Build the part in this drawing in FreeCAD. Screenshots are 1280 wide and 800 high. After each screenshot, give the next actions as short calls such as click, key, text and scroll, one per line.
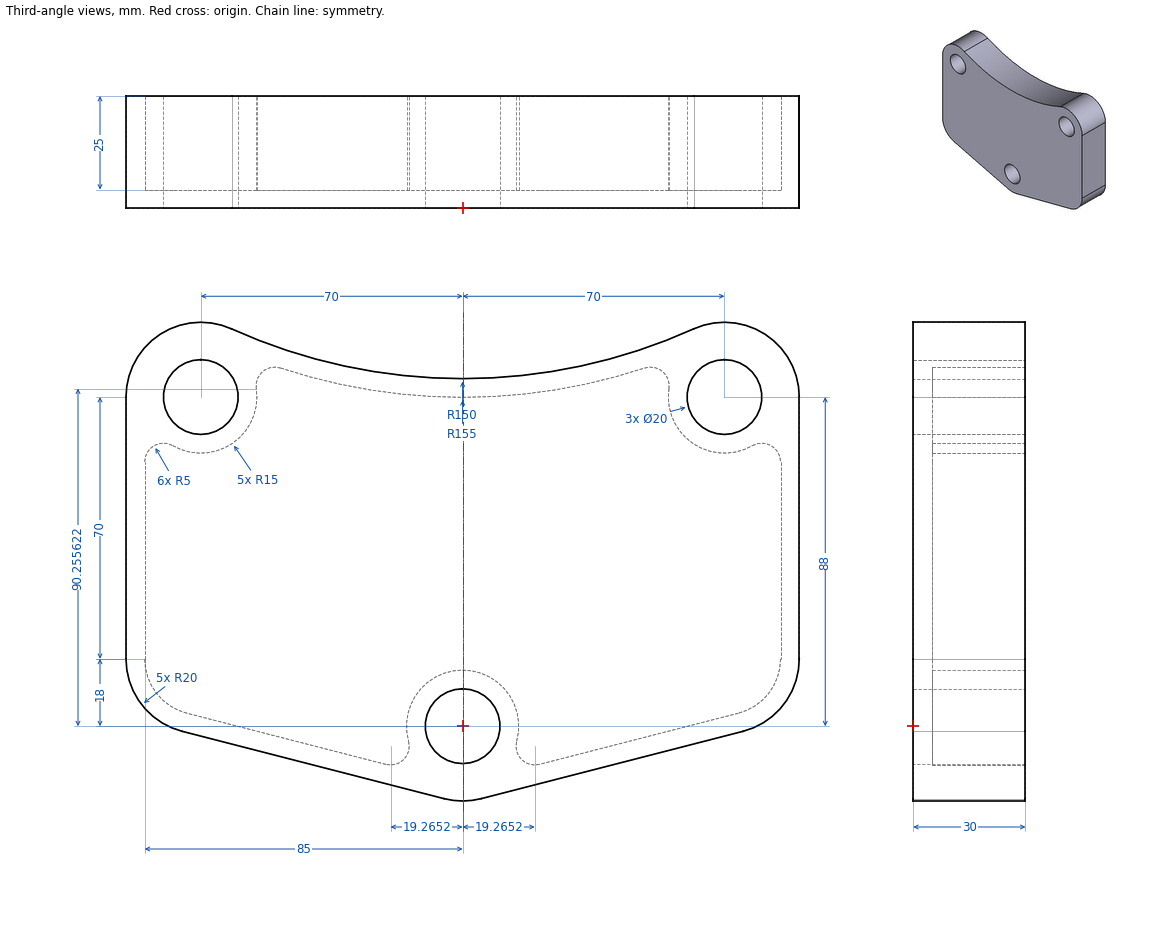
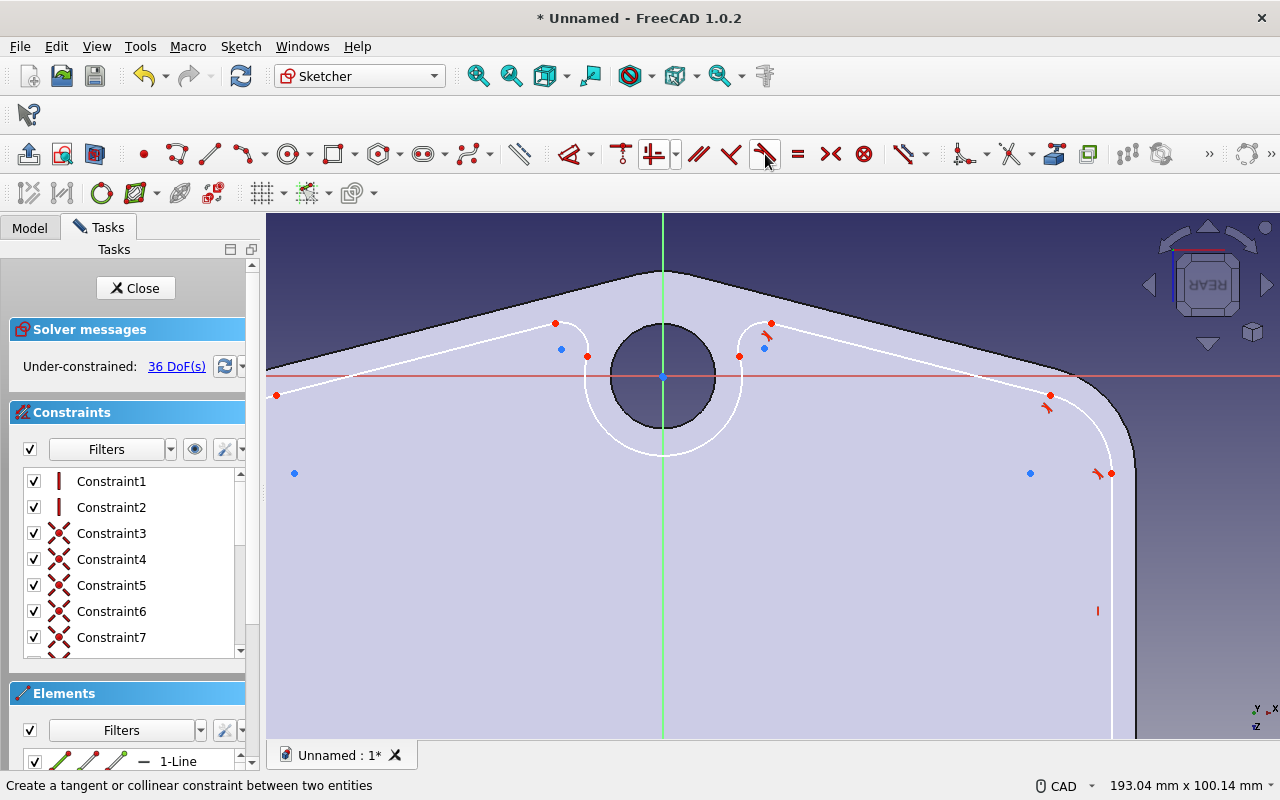
click(471, 345)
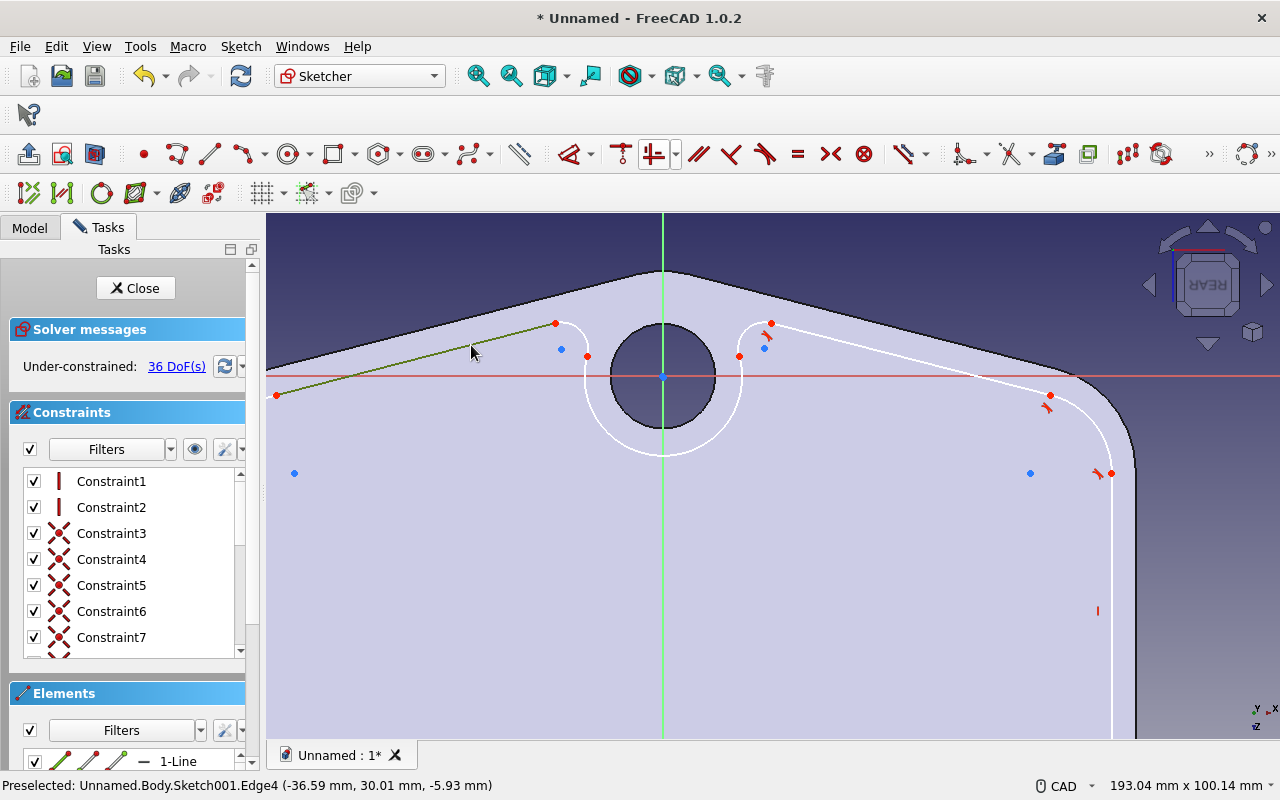
click(587, 340)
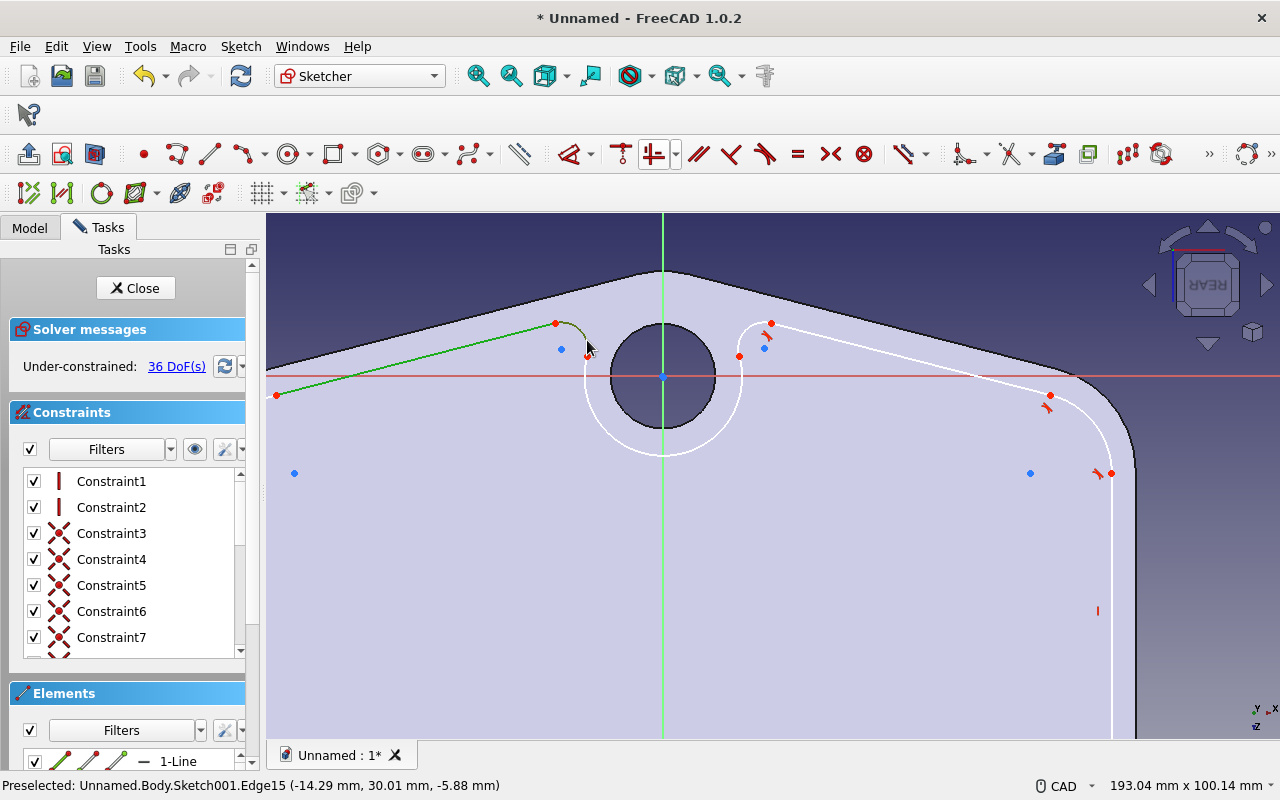
click(765, 154)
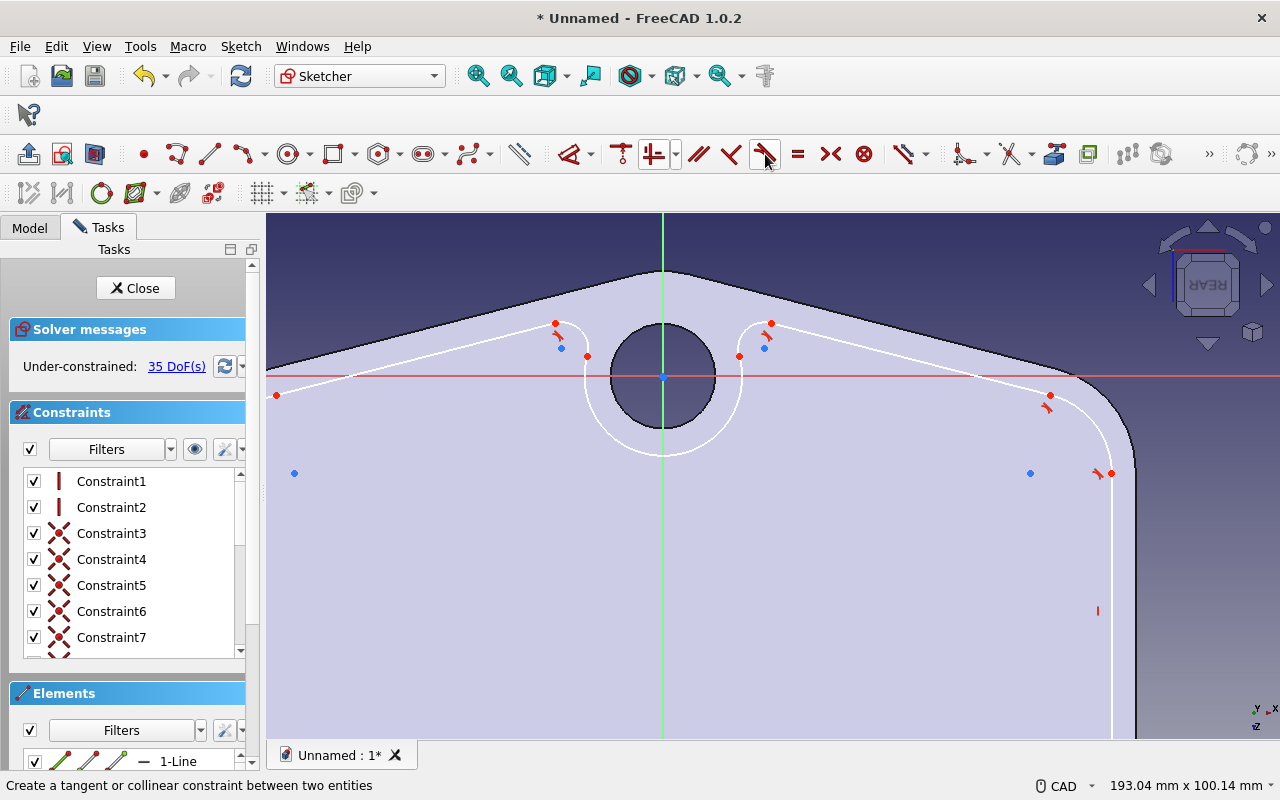
click(471, 345)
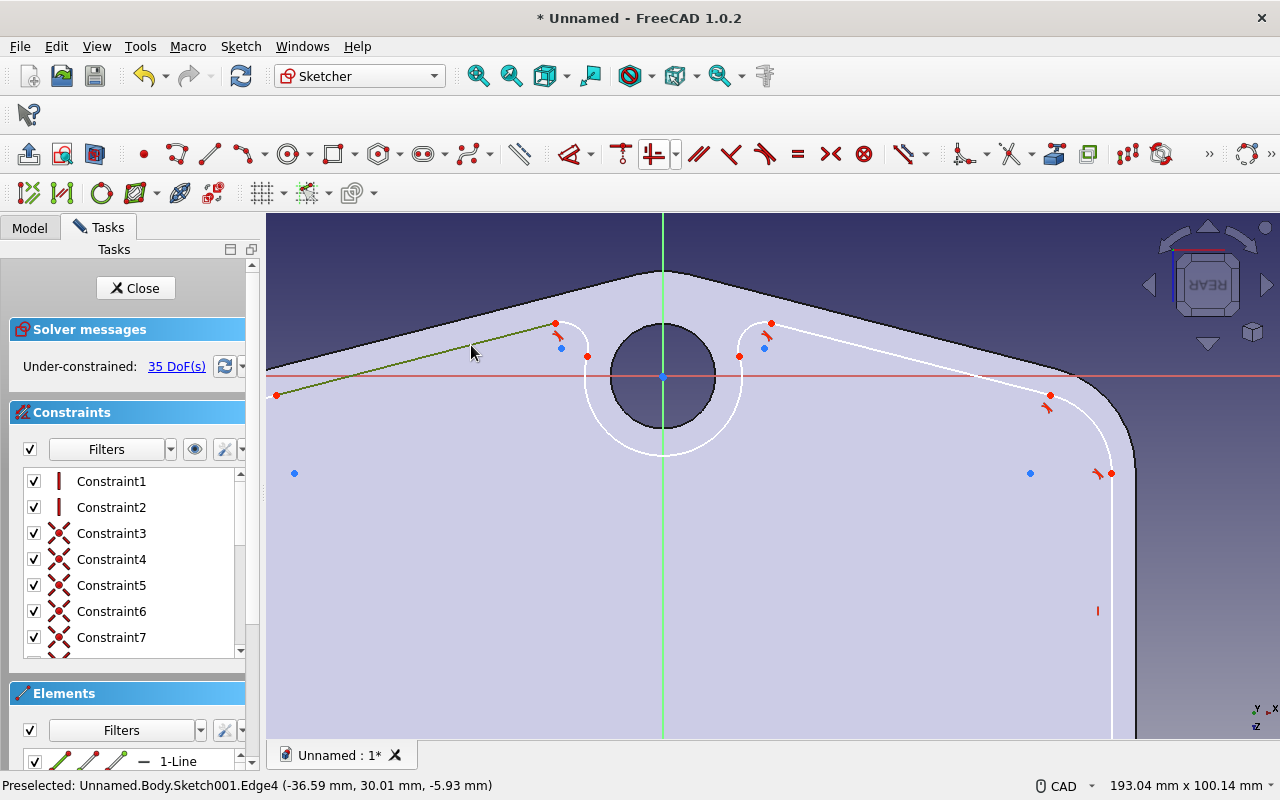
scroll(755, 324, down, 3)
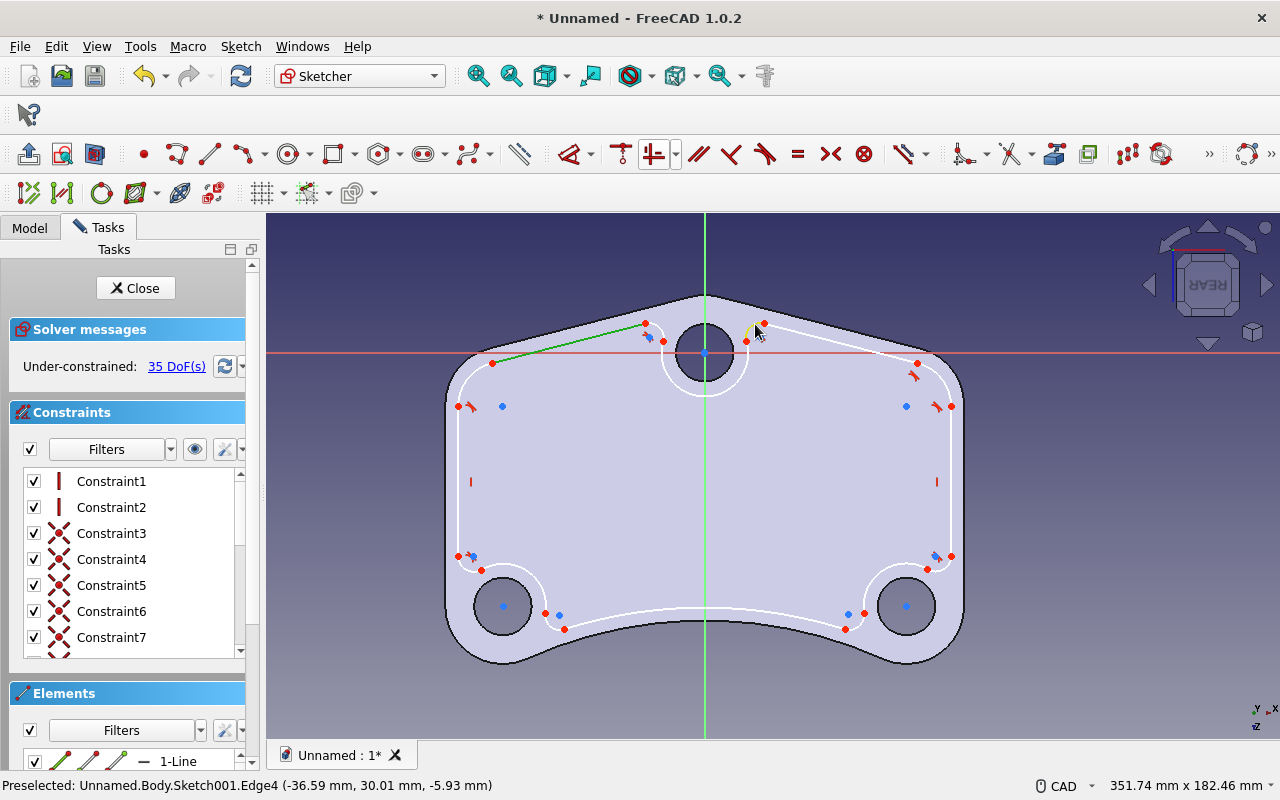
click(476, 371)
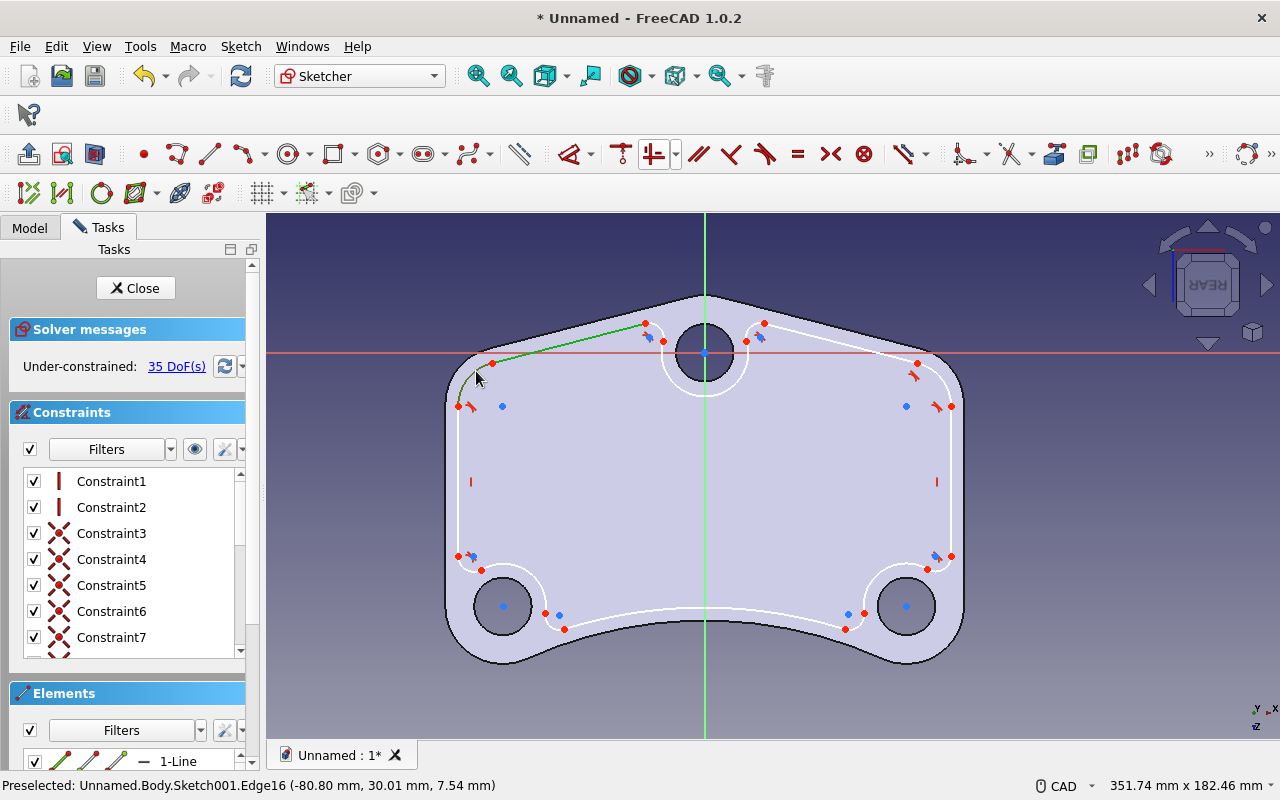
click(765, 154)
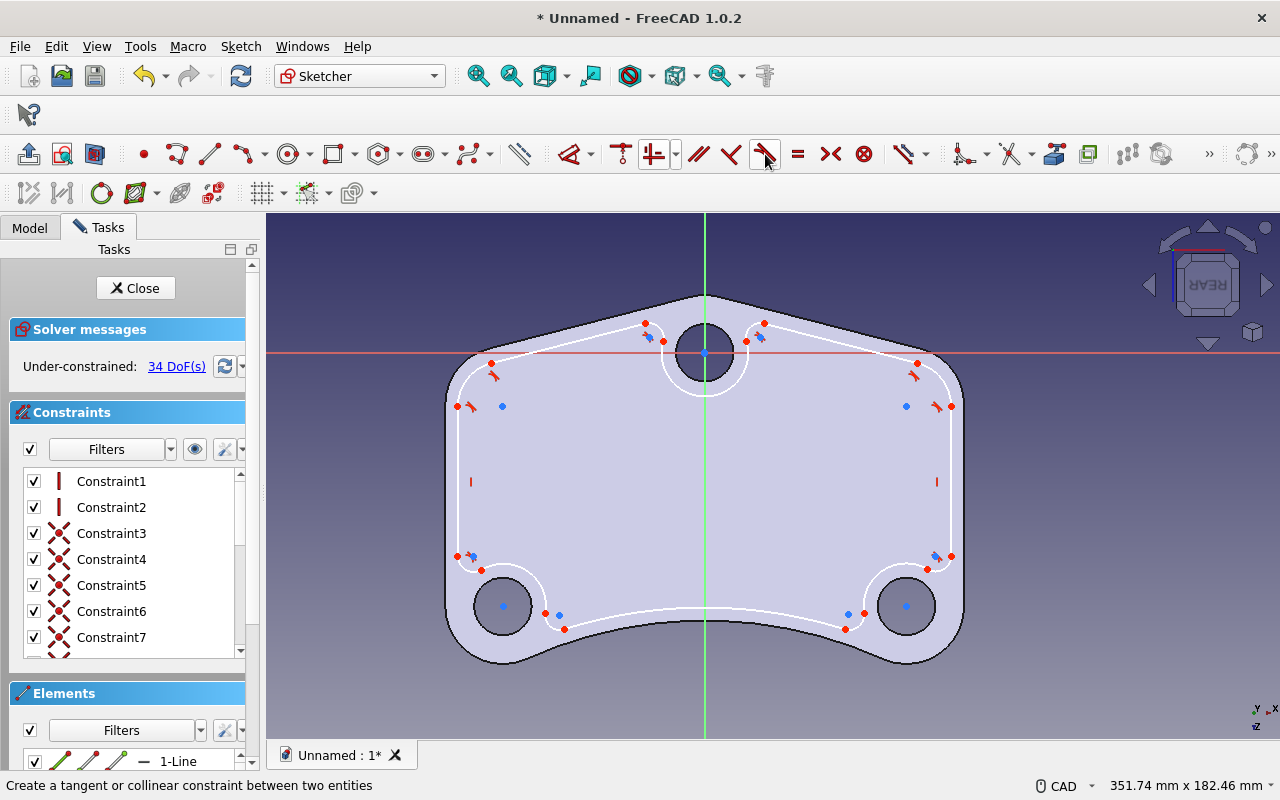
scroll(461, 565, up, 2)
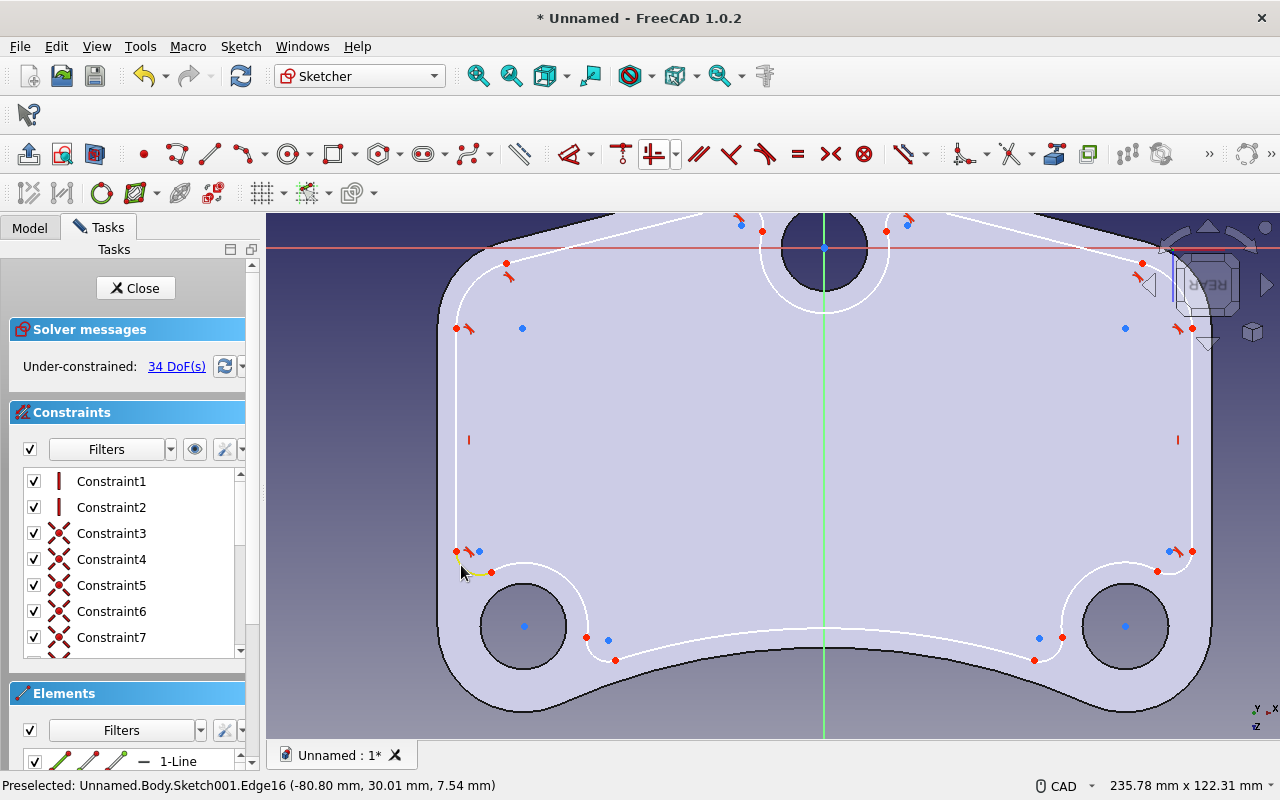
click(461, 565)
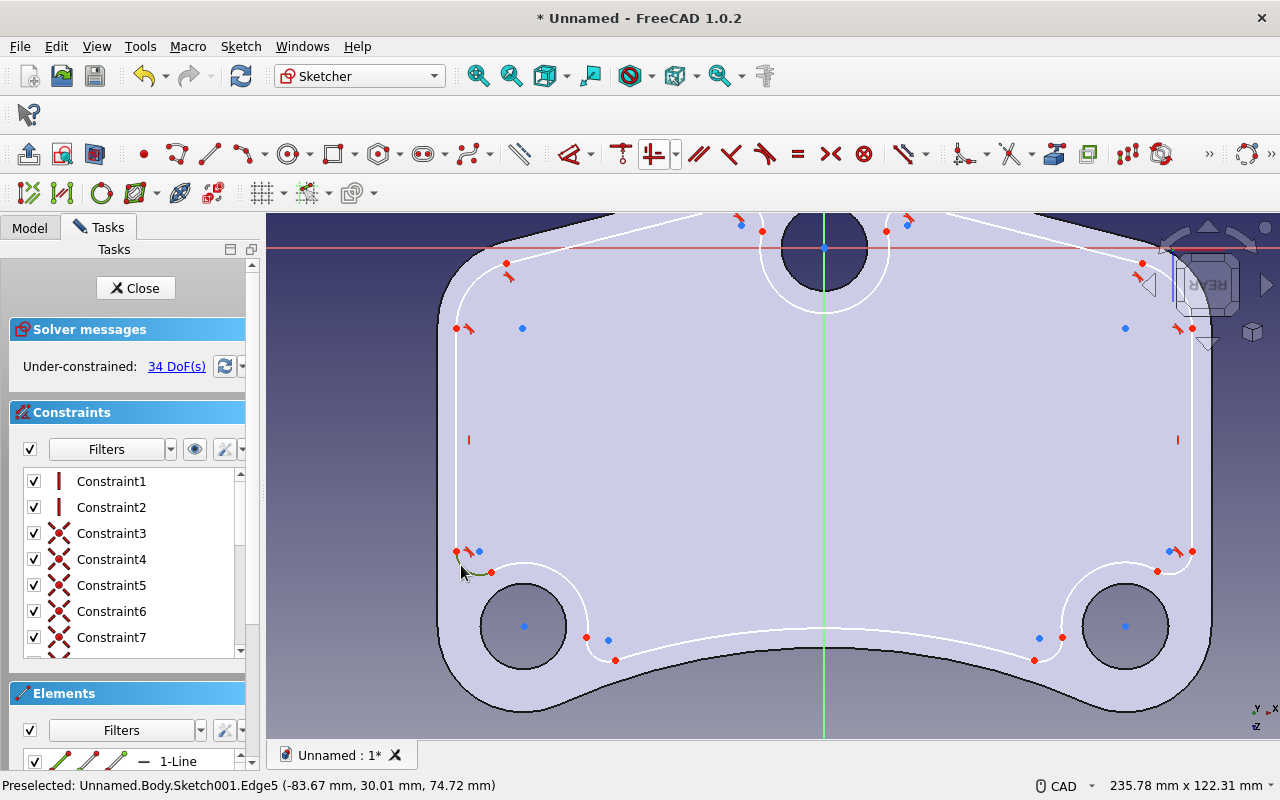
click(579, 595)